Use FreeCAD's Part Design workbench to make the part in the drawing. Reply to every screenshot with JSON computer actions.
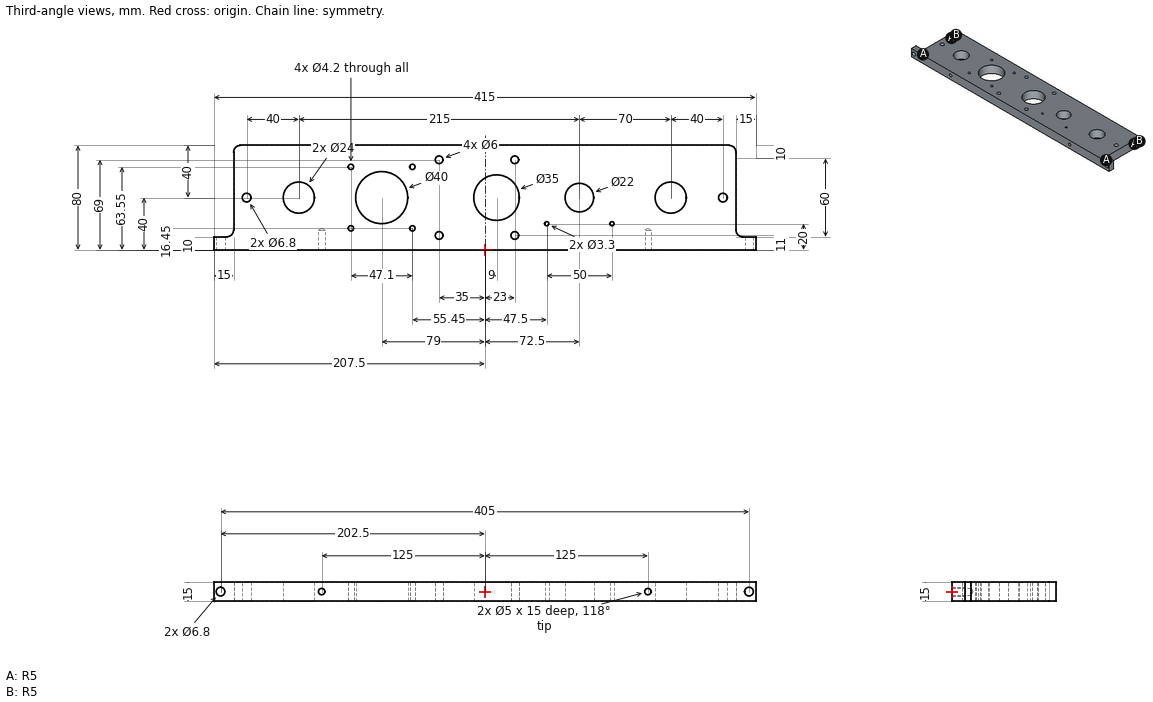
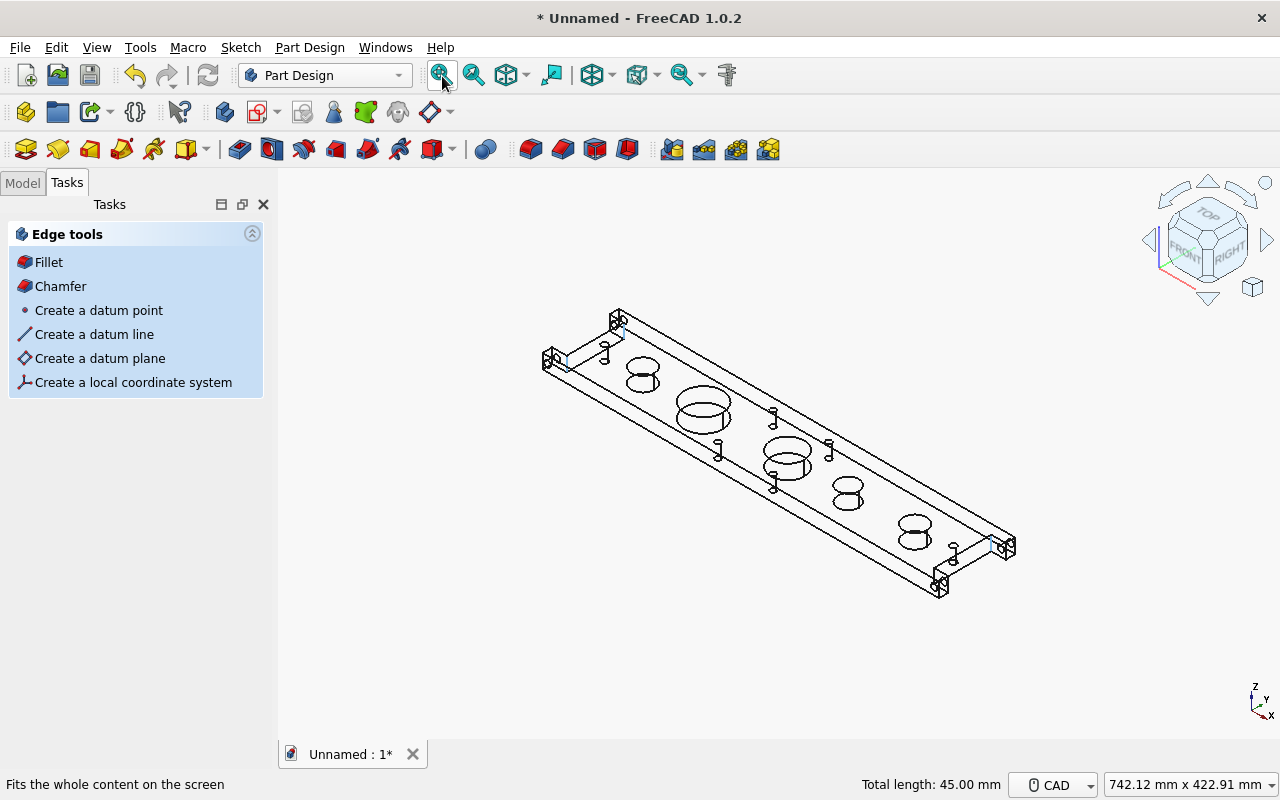
{"action": "key", "text": "2"}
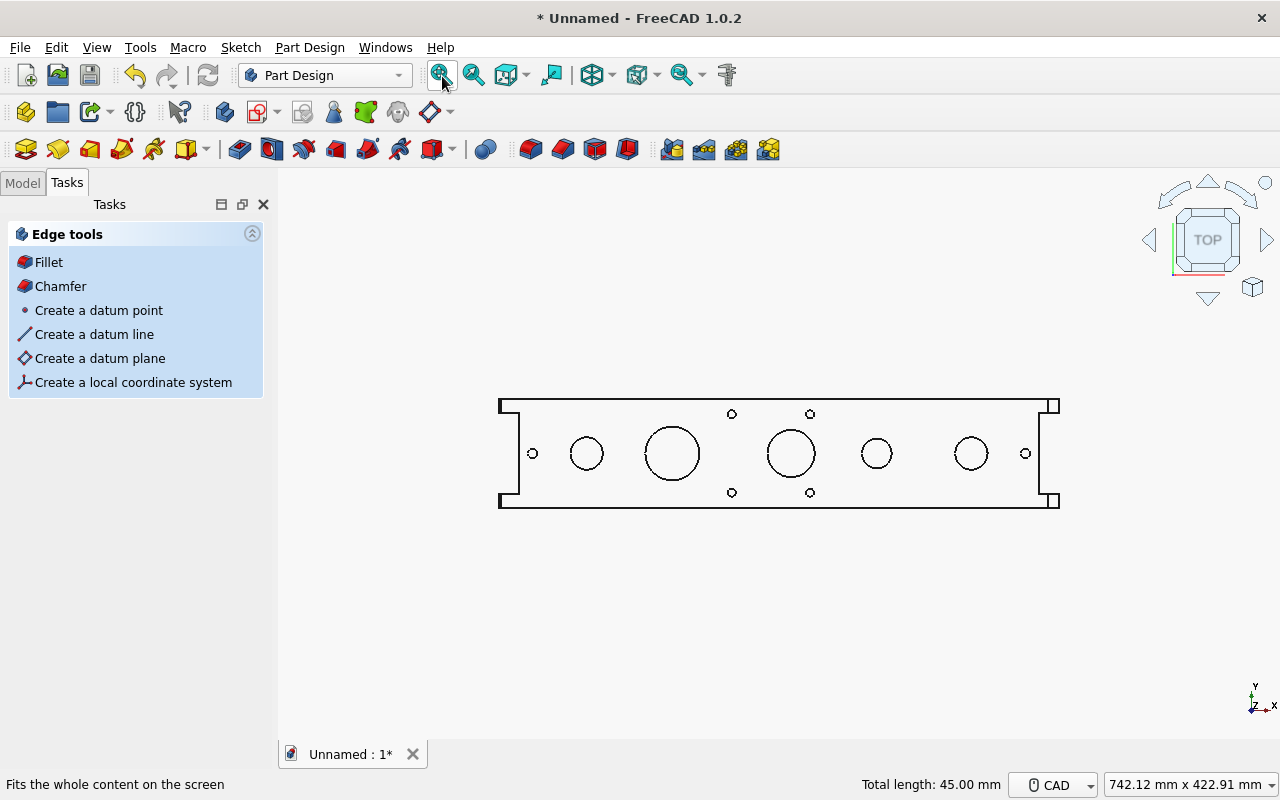
{"action": "scroll", "coordinate": [1039, 493], "scroll_direction": "up", "scroll_amount": 6}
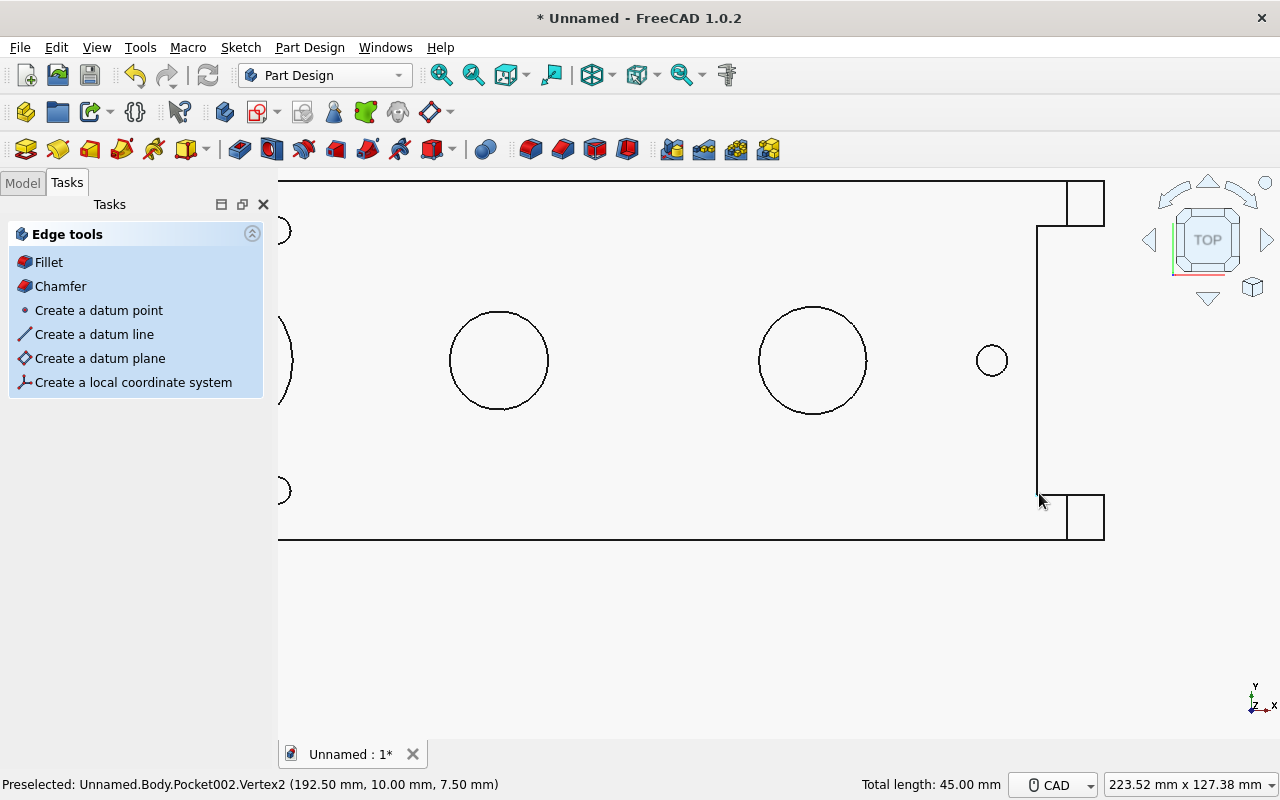
{"action": "left_click", "coordinate": [442, 76]}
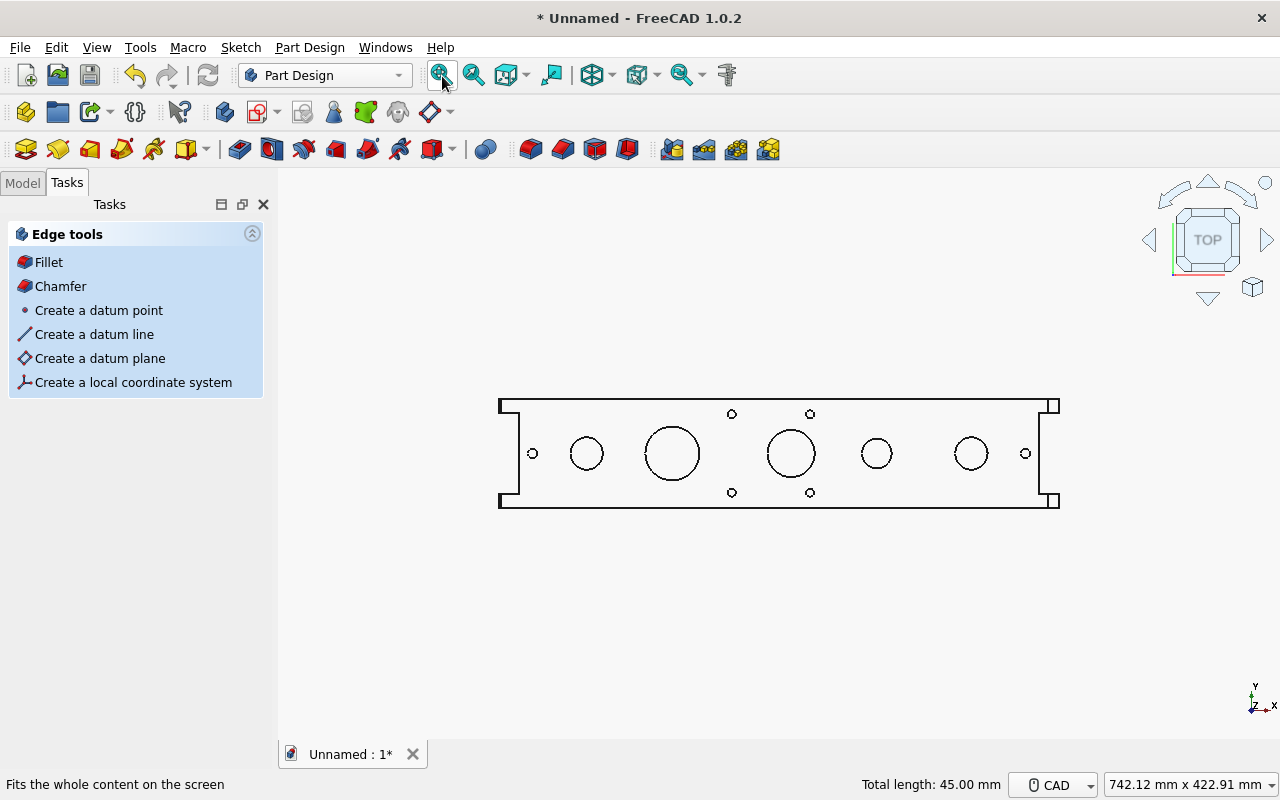
{"action": "key", "text": "1"}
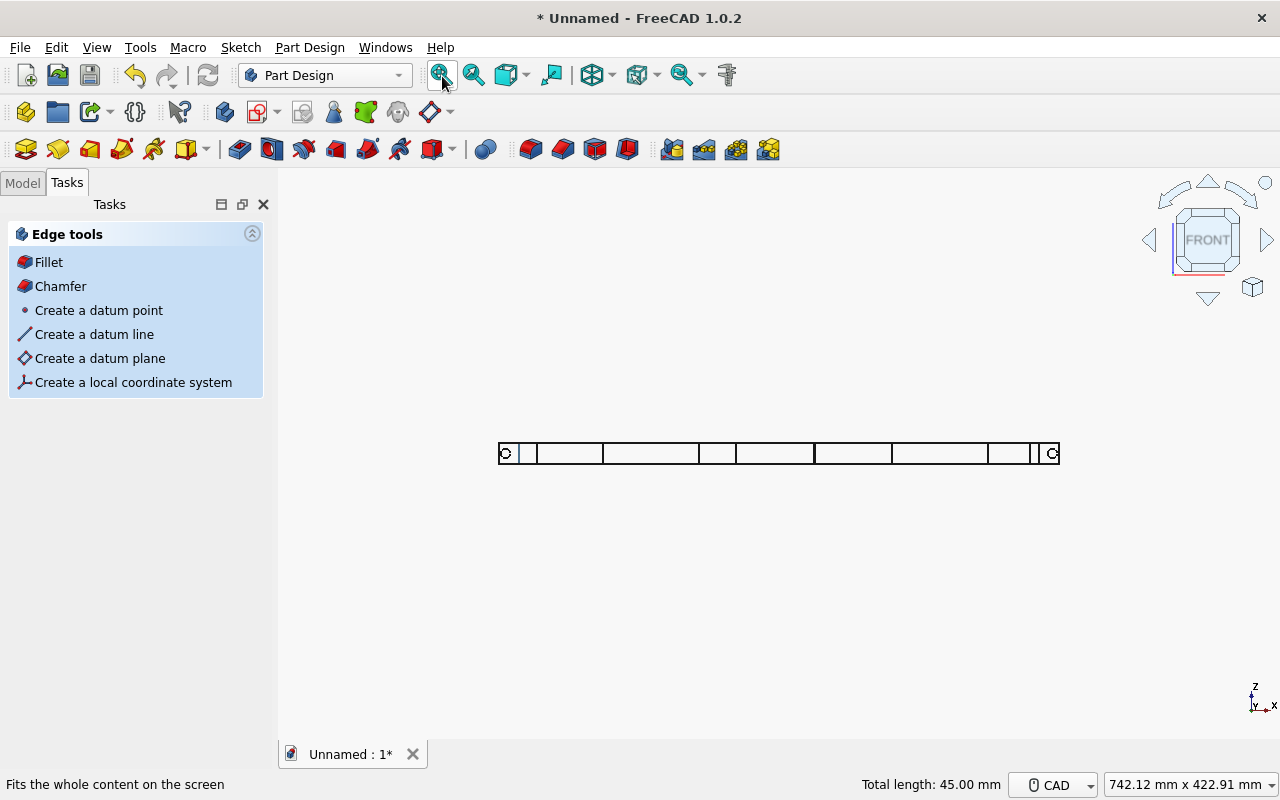
{"action": "left_click", "coordinate": [1039, 452], "text": "ctrl"}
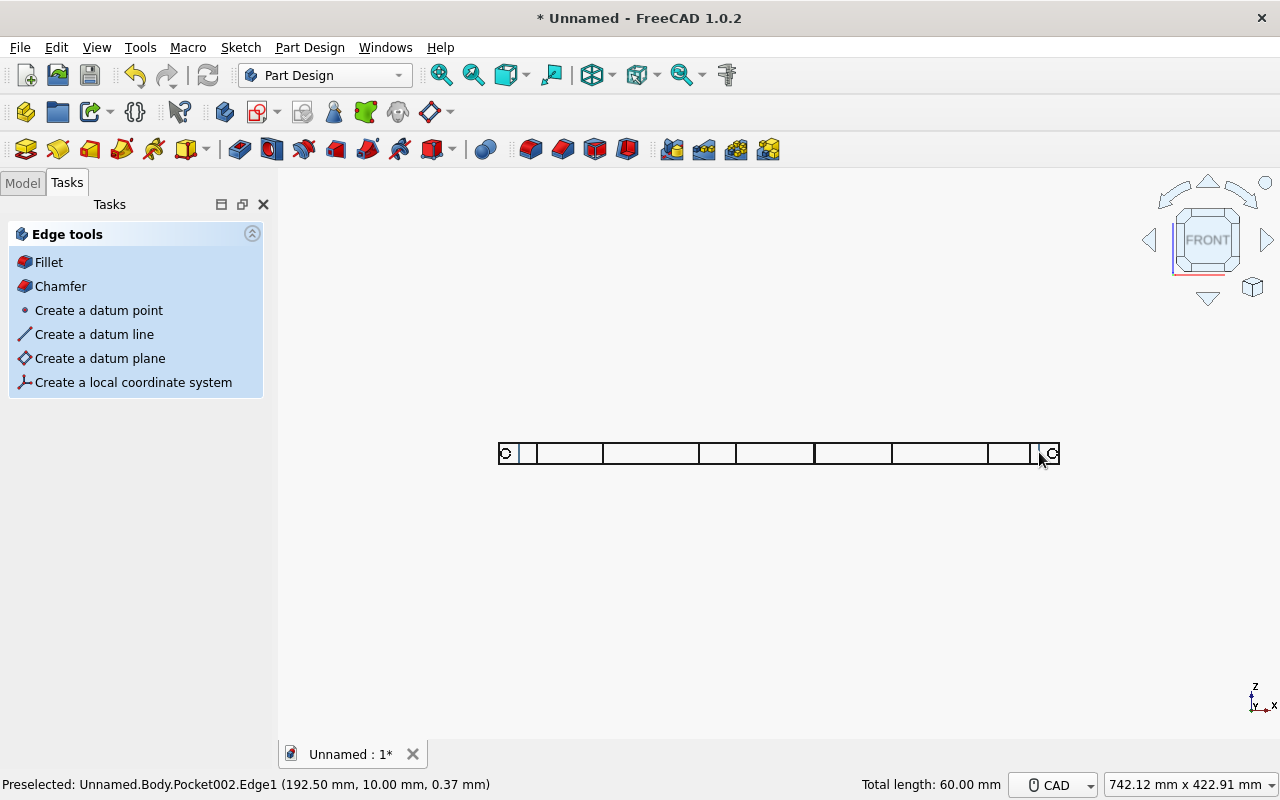
{"action": "key", "text": "v 1"}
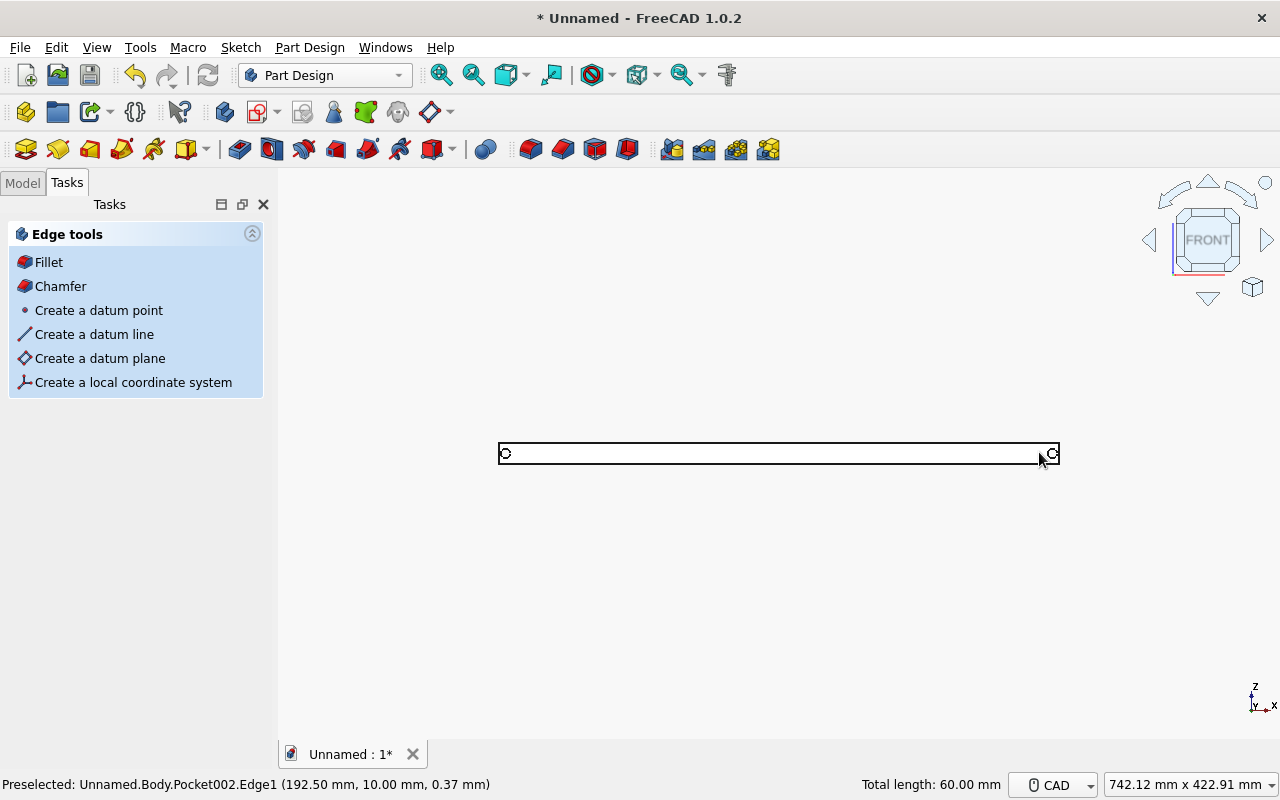
{"action": "left_click", "coordinate": [532, 150]}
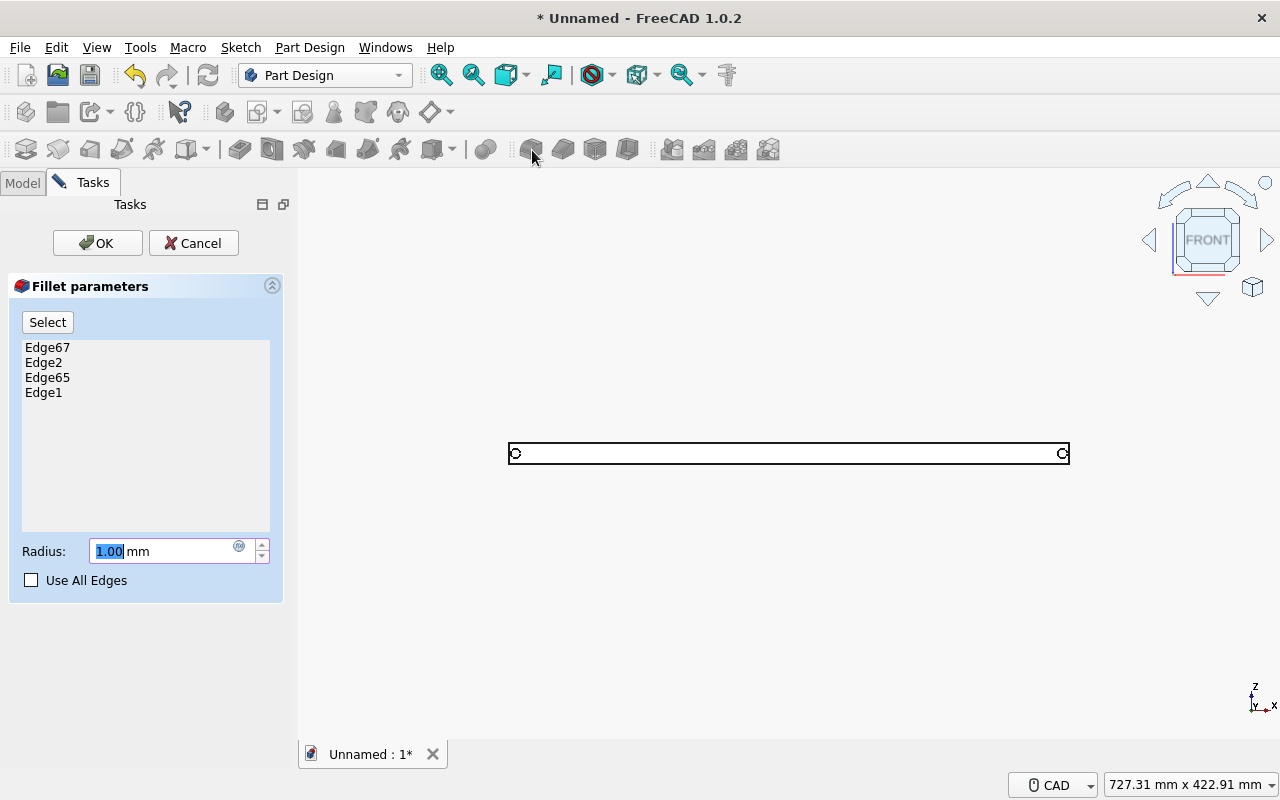
{"action": "type", "text": "5"}
{"action": "key", "text": "Tab"}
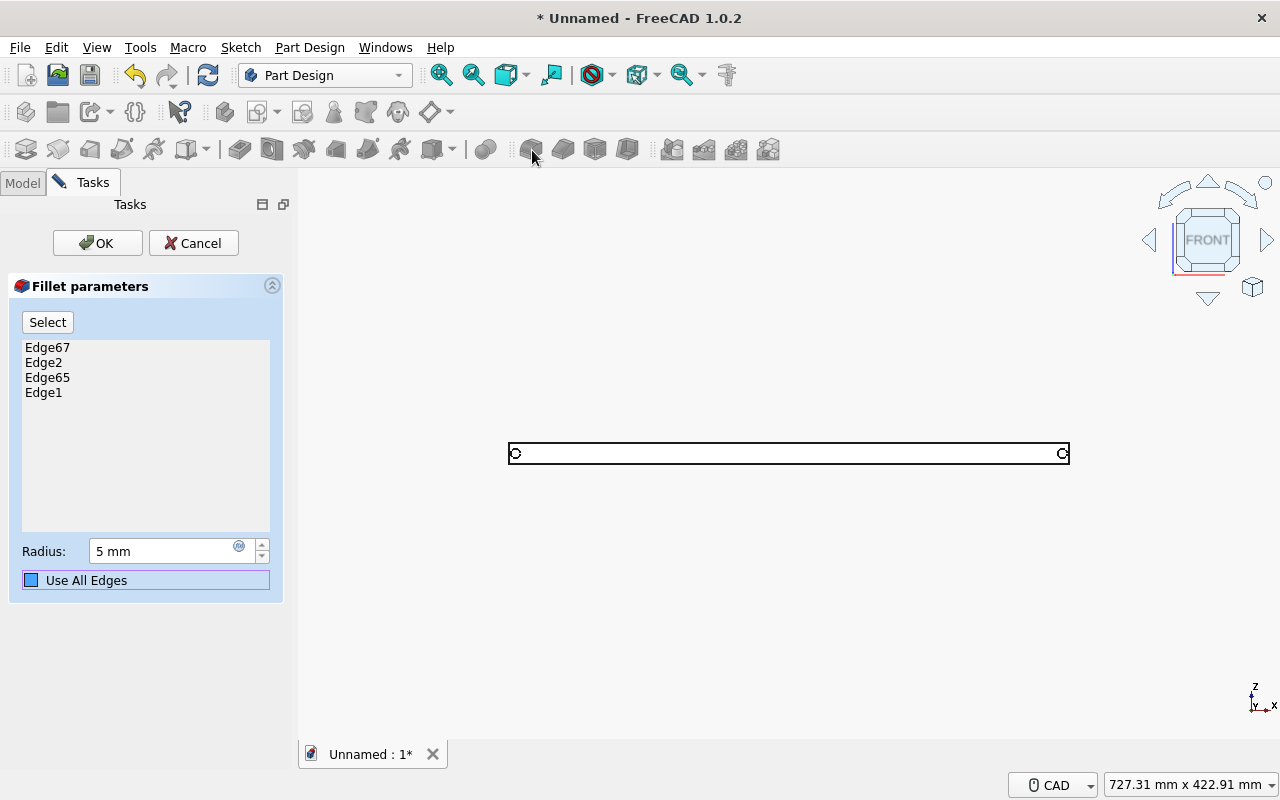
{"action": "left_click", "coordinate": [98, 243]}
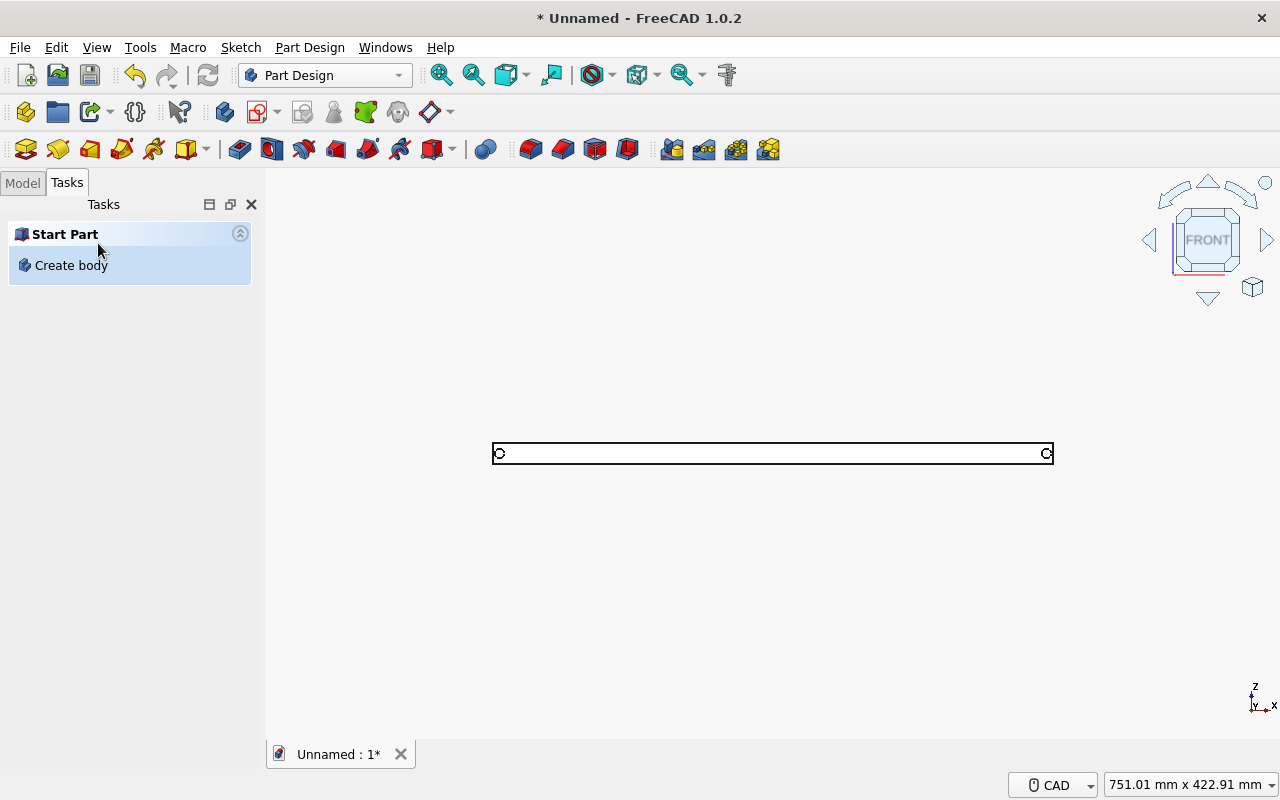
{"action": "key", "text": "0"}